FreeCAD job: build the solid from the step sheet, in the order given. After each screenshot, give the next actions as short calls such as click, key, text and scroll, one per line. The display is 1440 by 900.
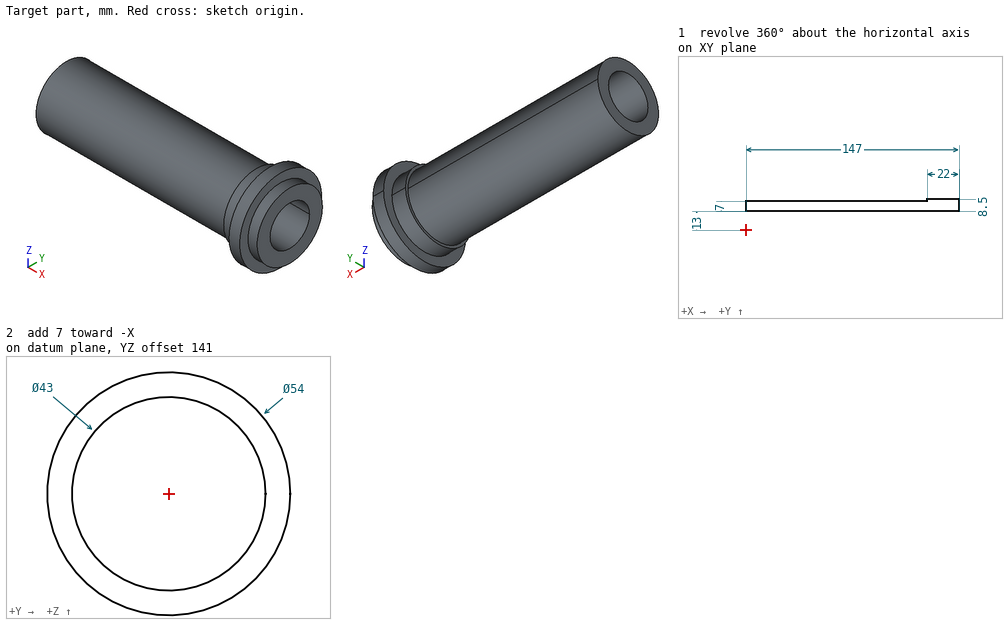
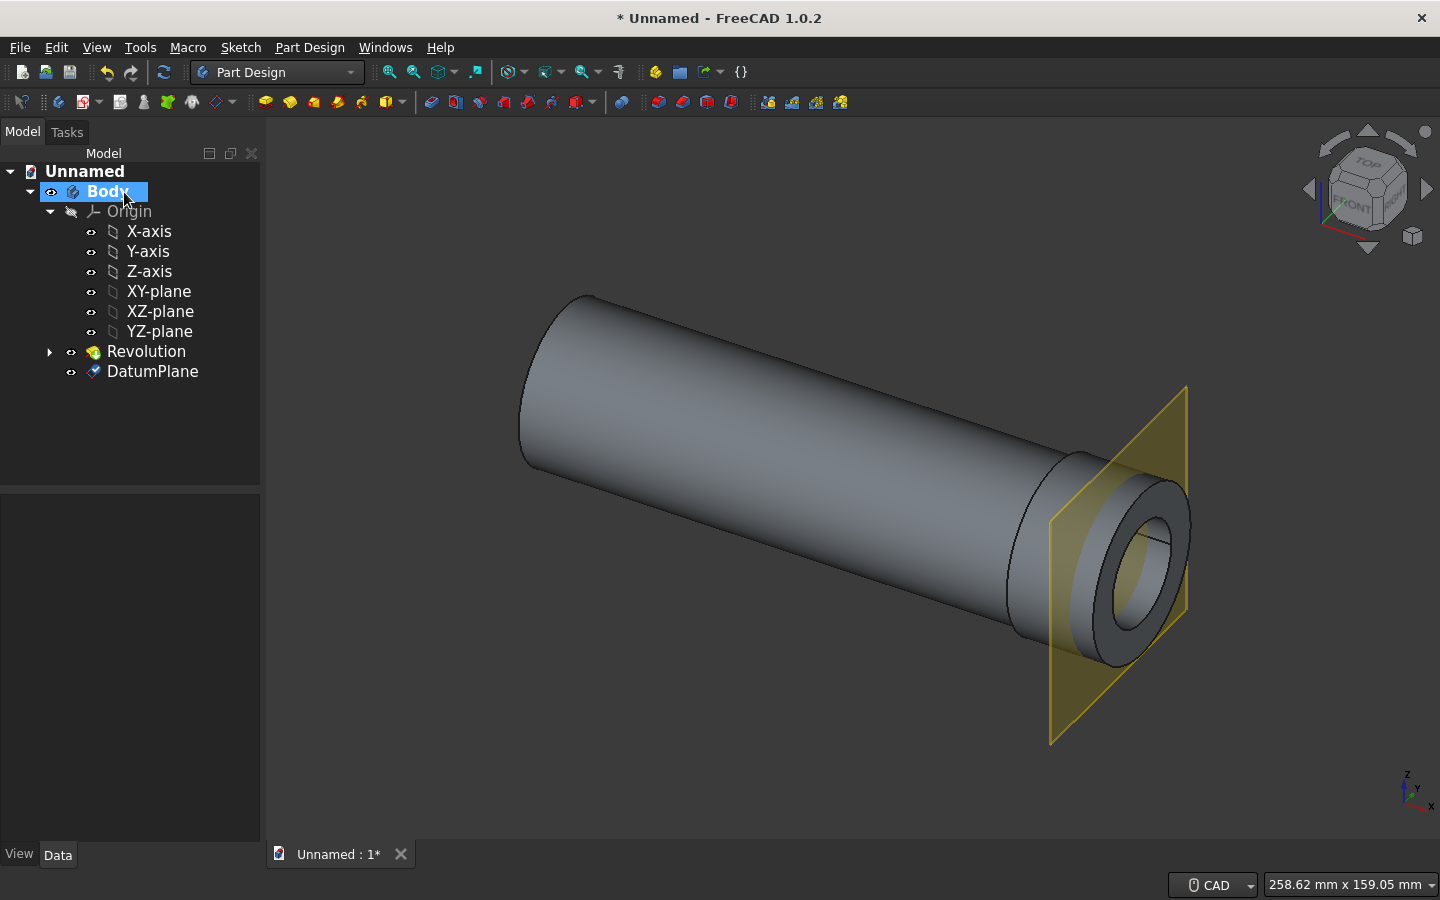
click(116, 372)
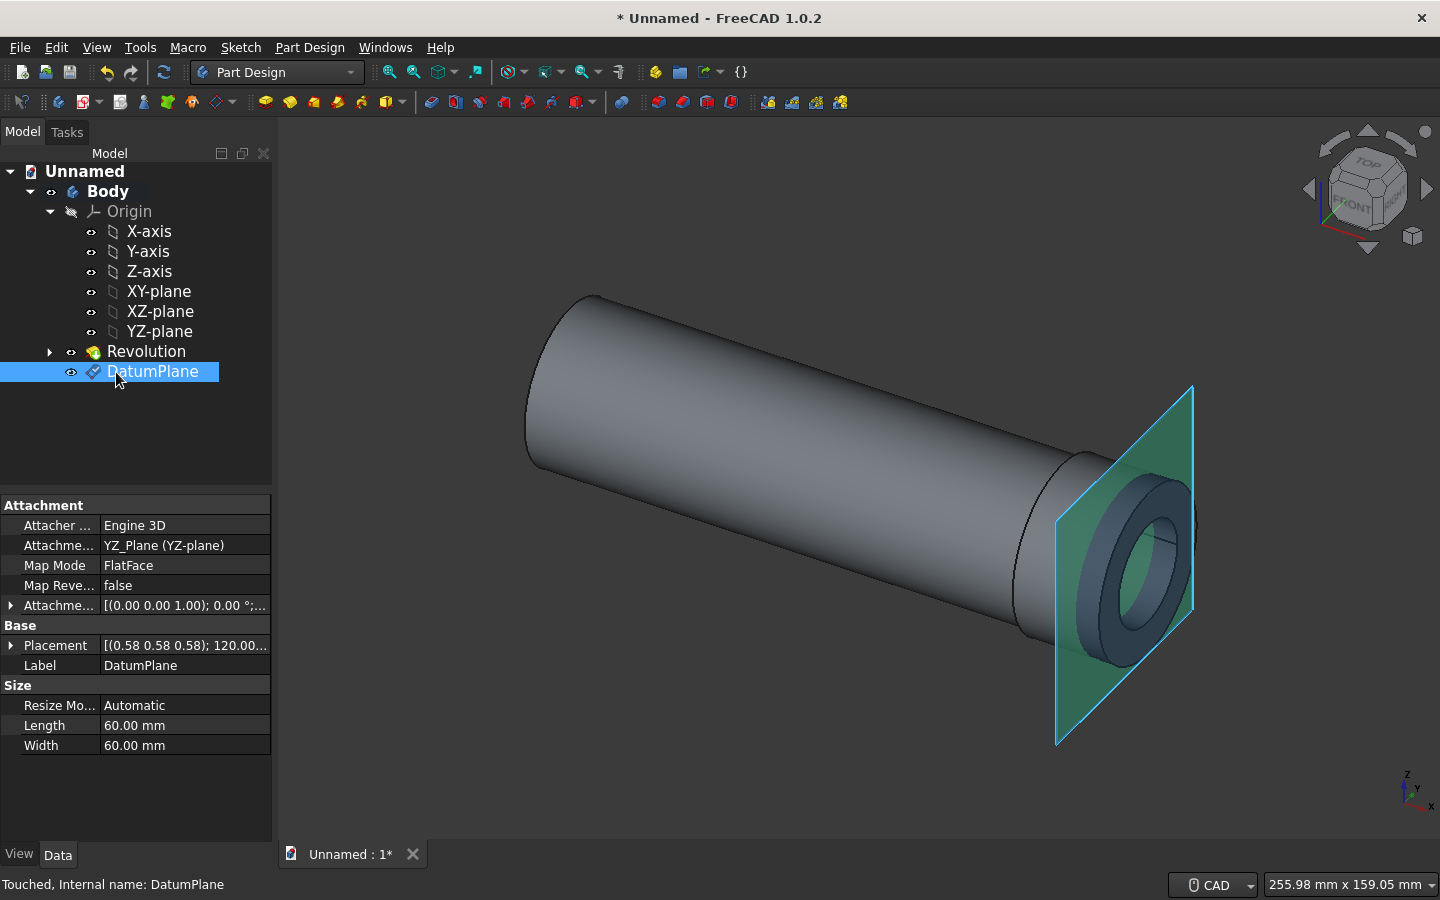
click(84, 102)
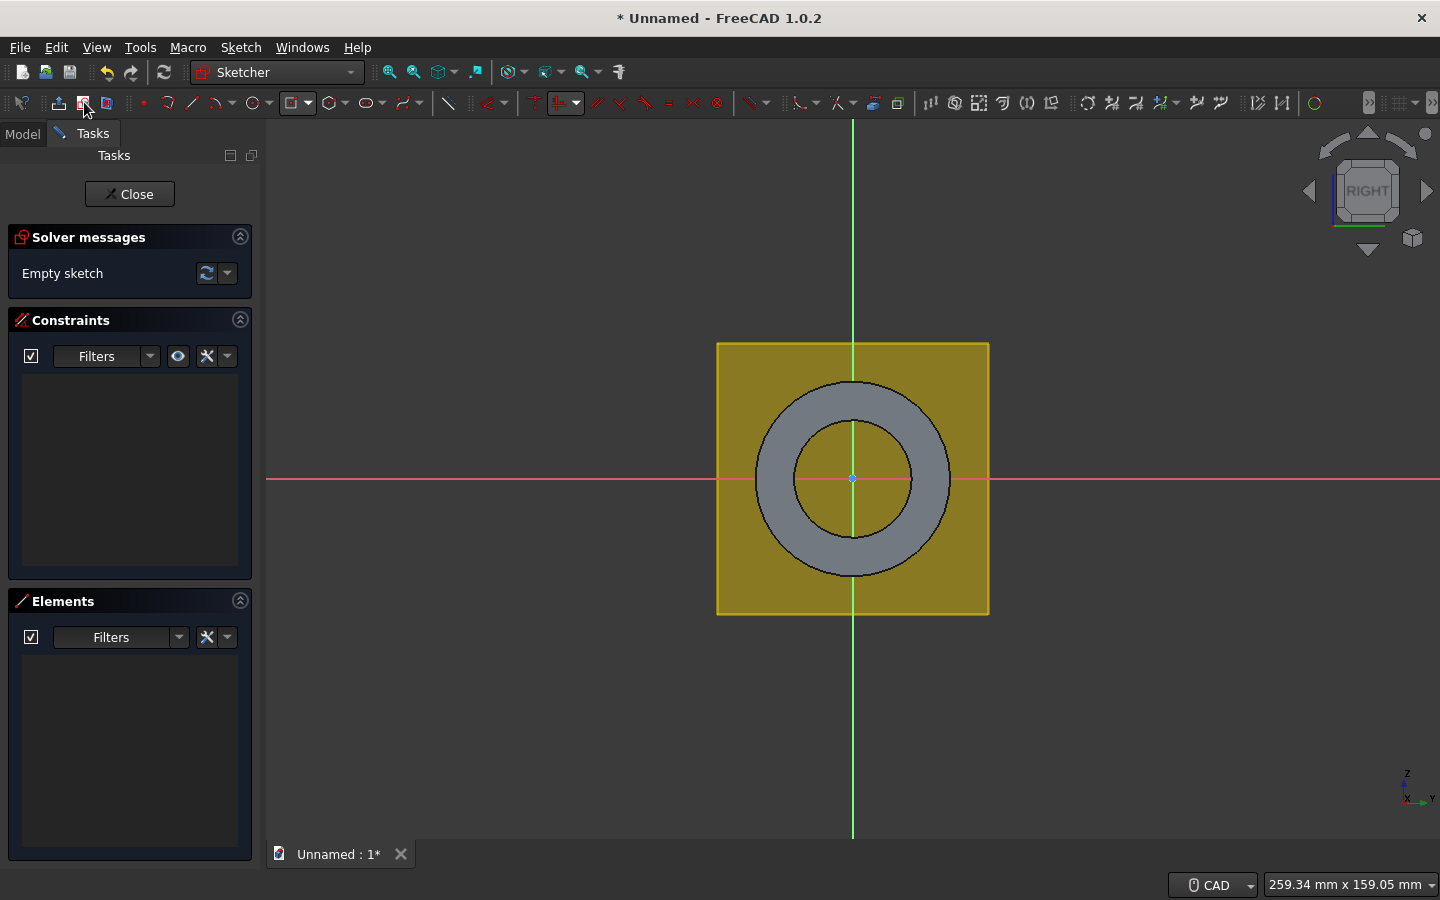
click(108, 104)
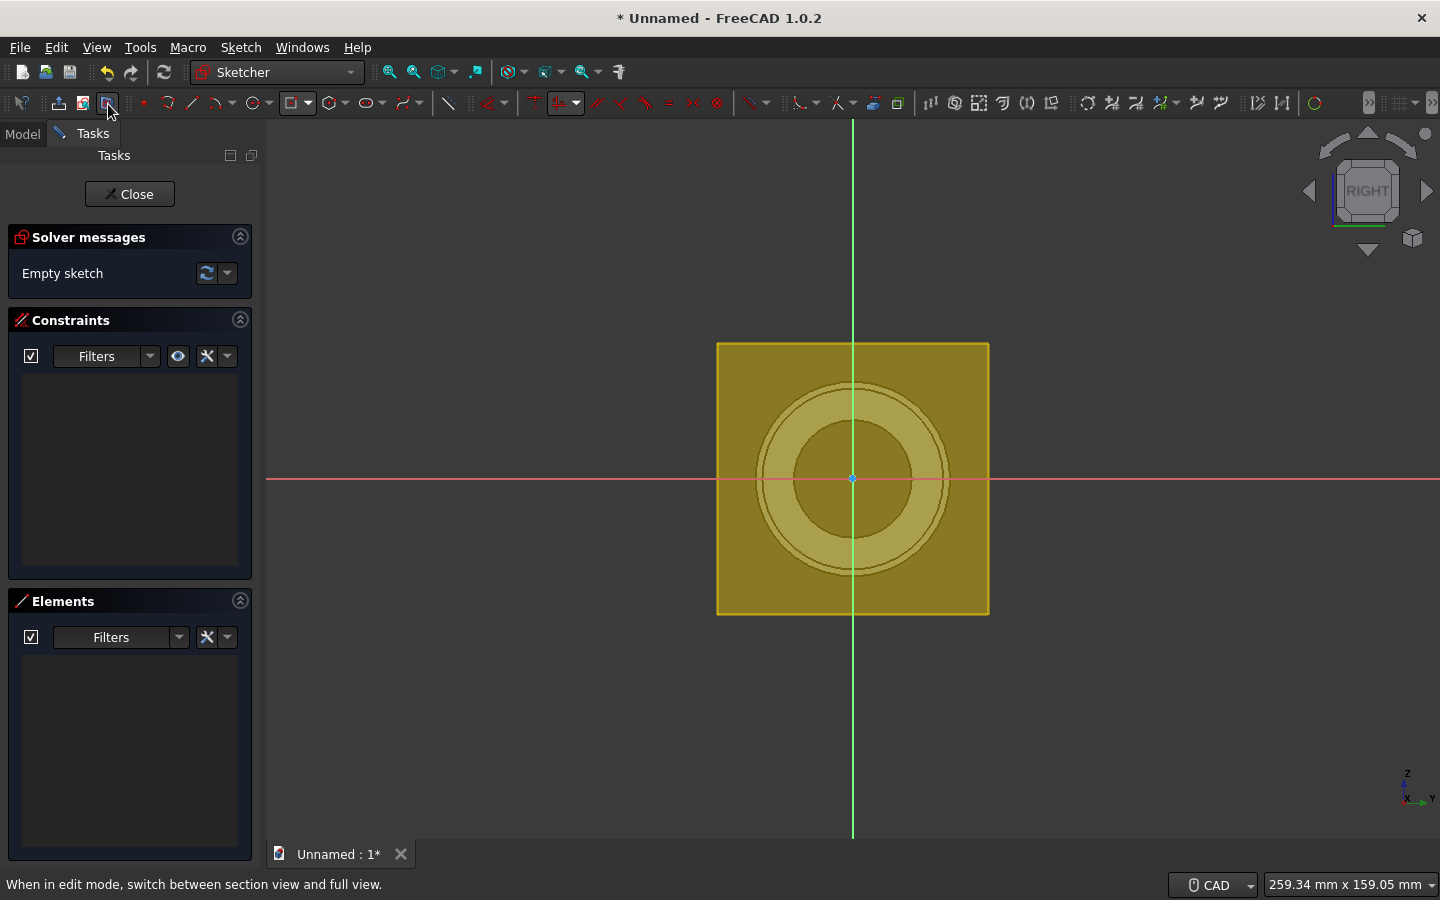
scroll(936, 479, up, 3)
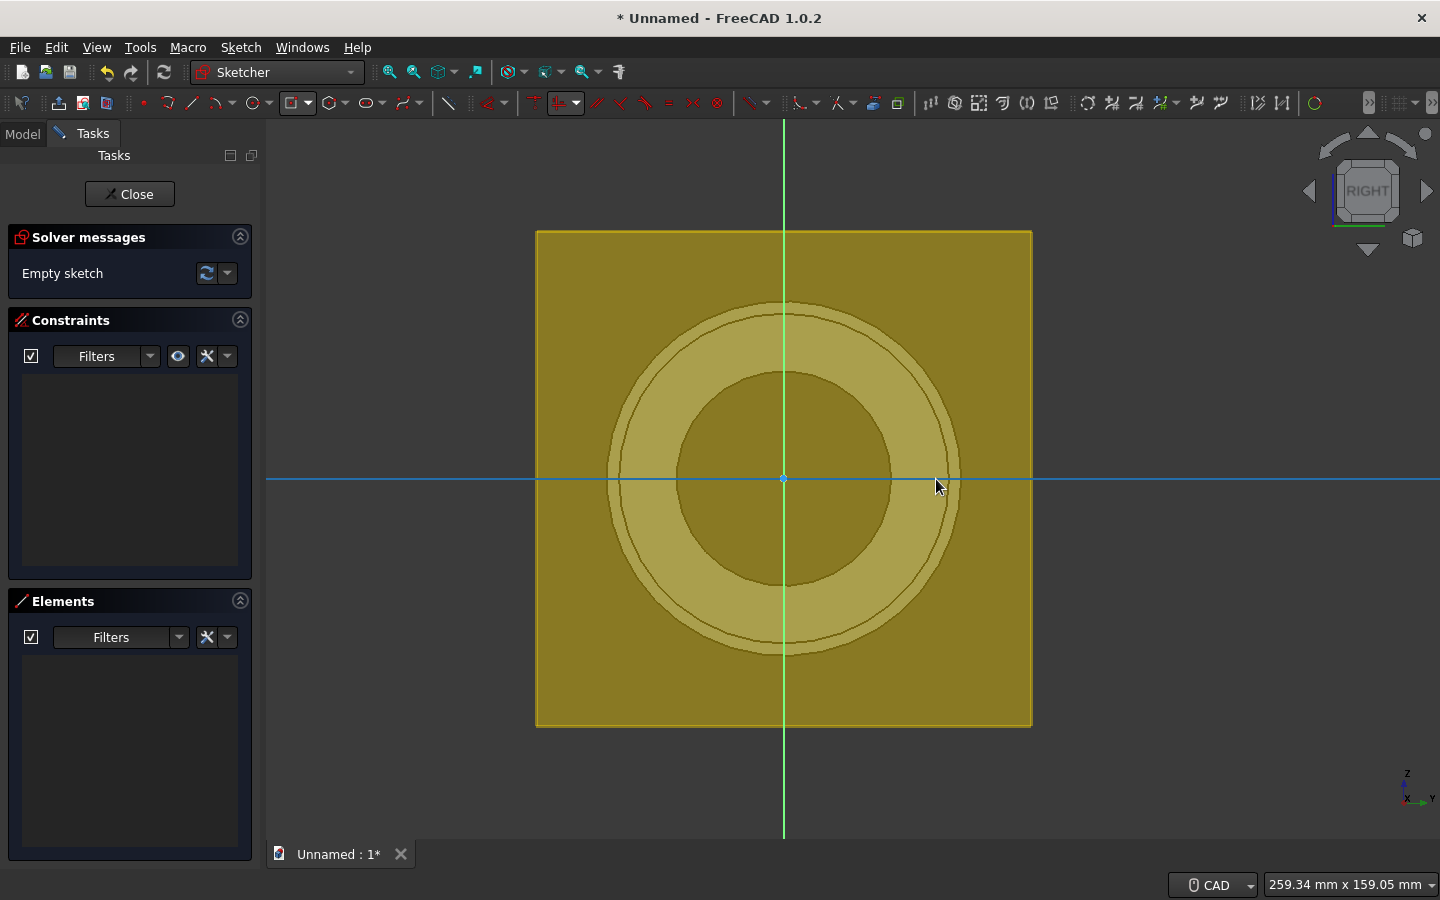
click(254, 104)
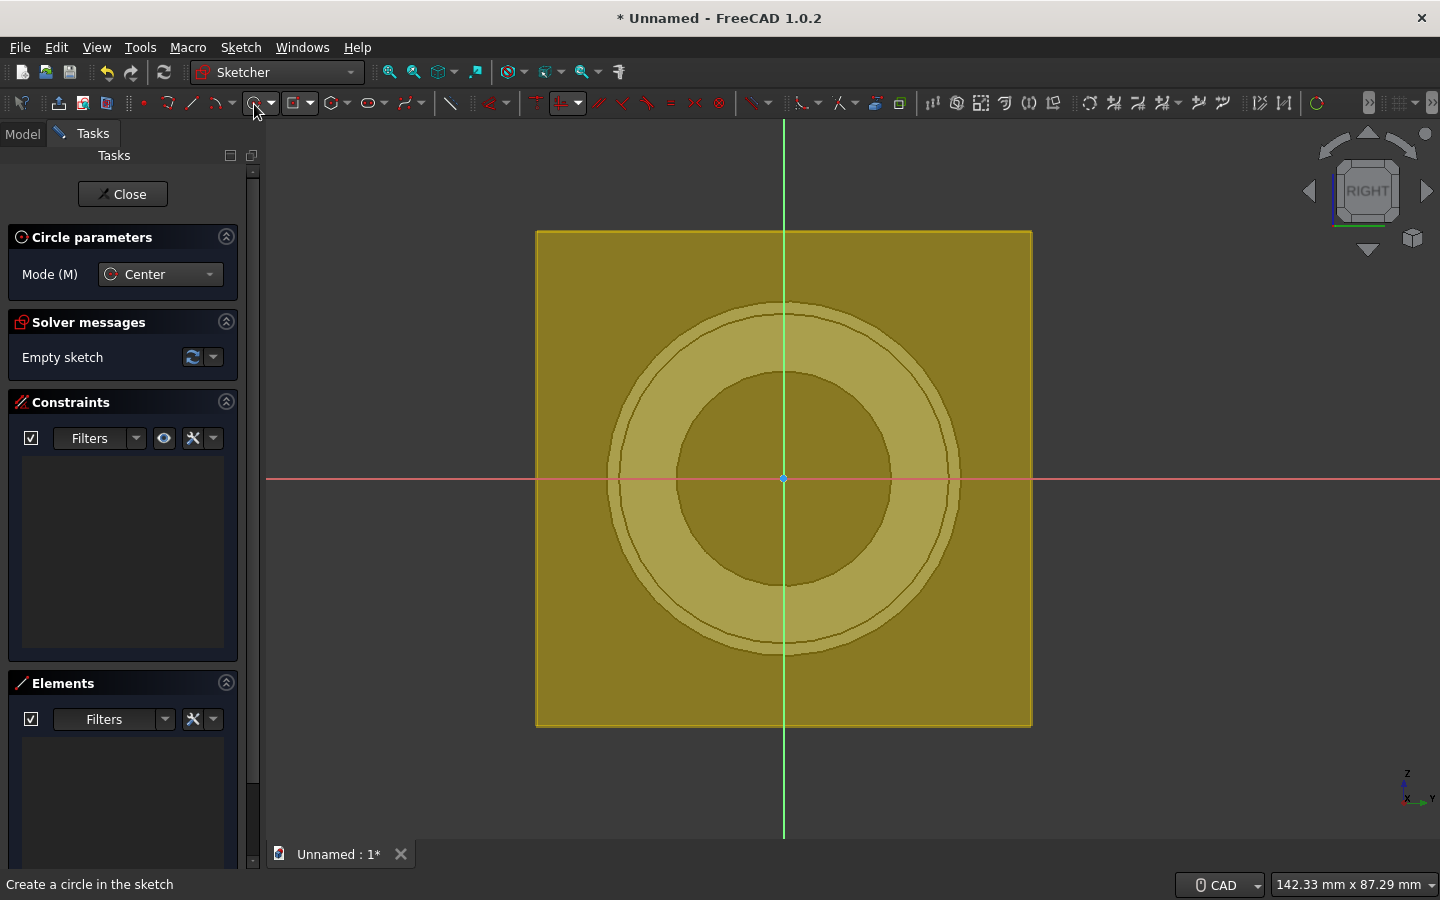
click(784, 479)
click(941, 321)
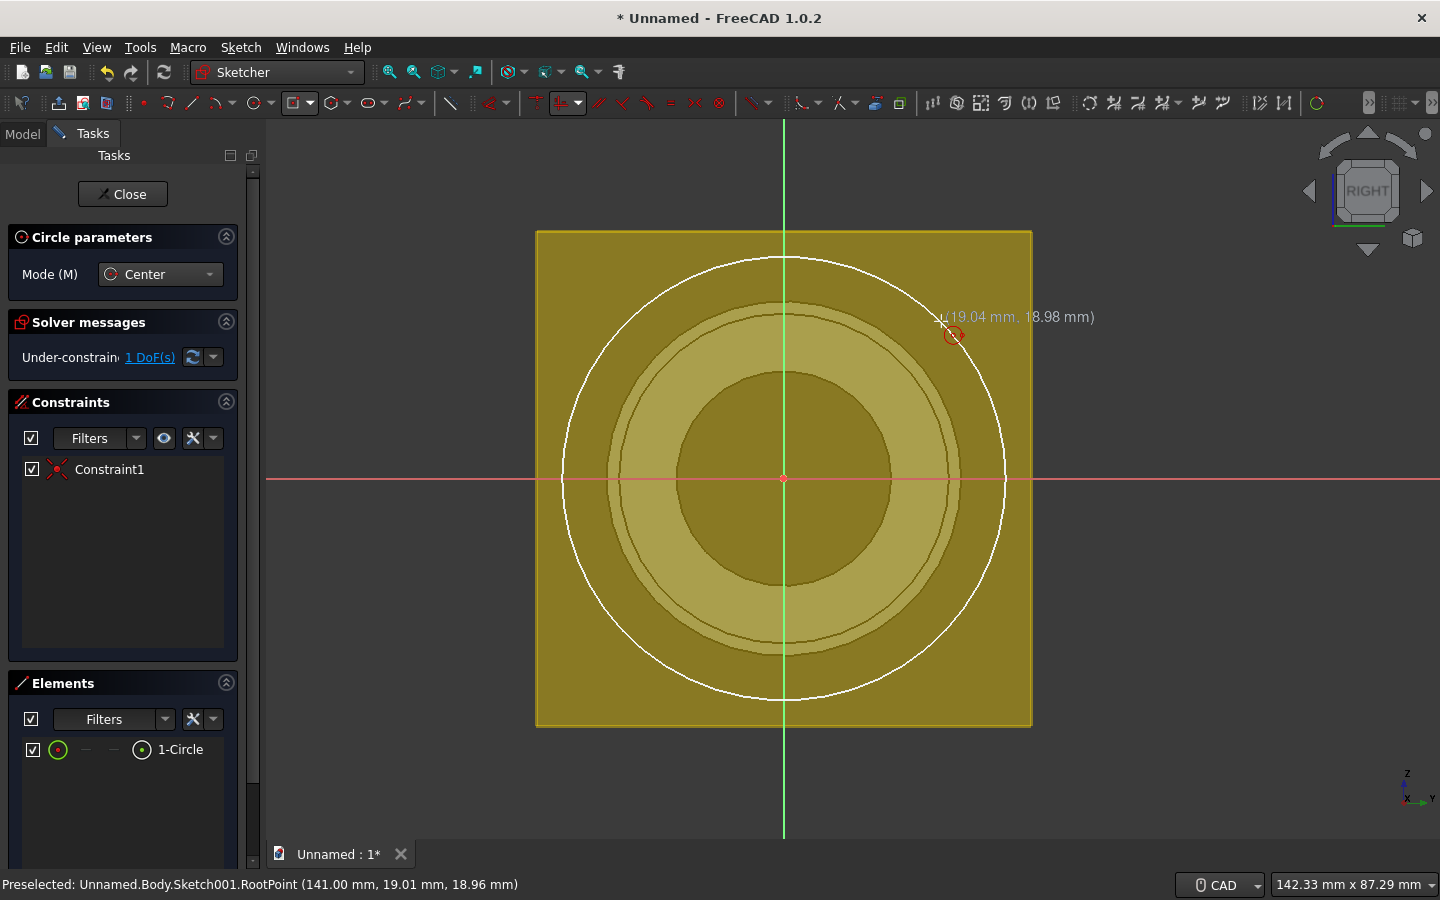
click(784, 479)
click(909, 353)
key(Escape)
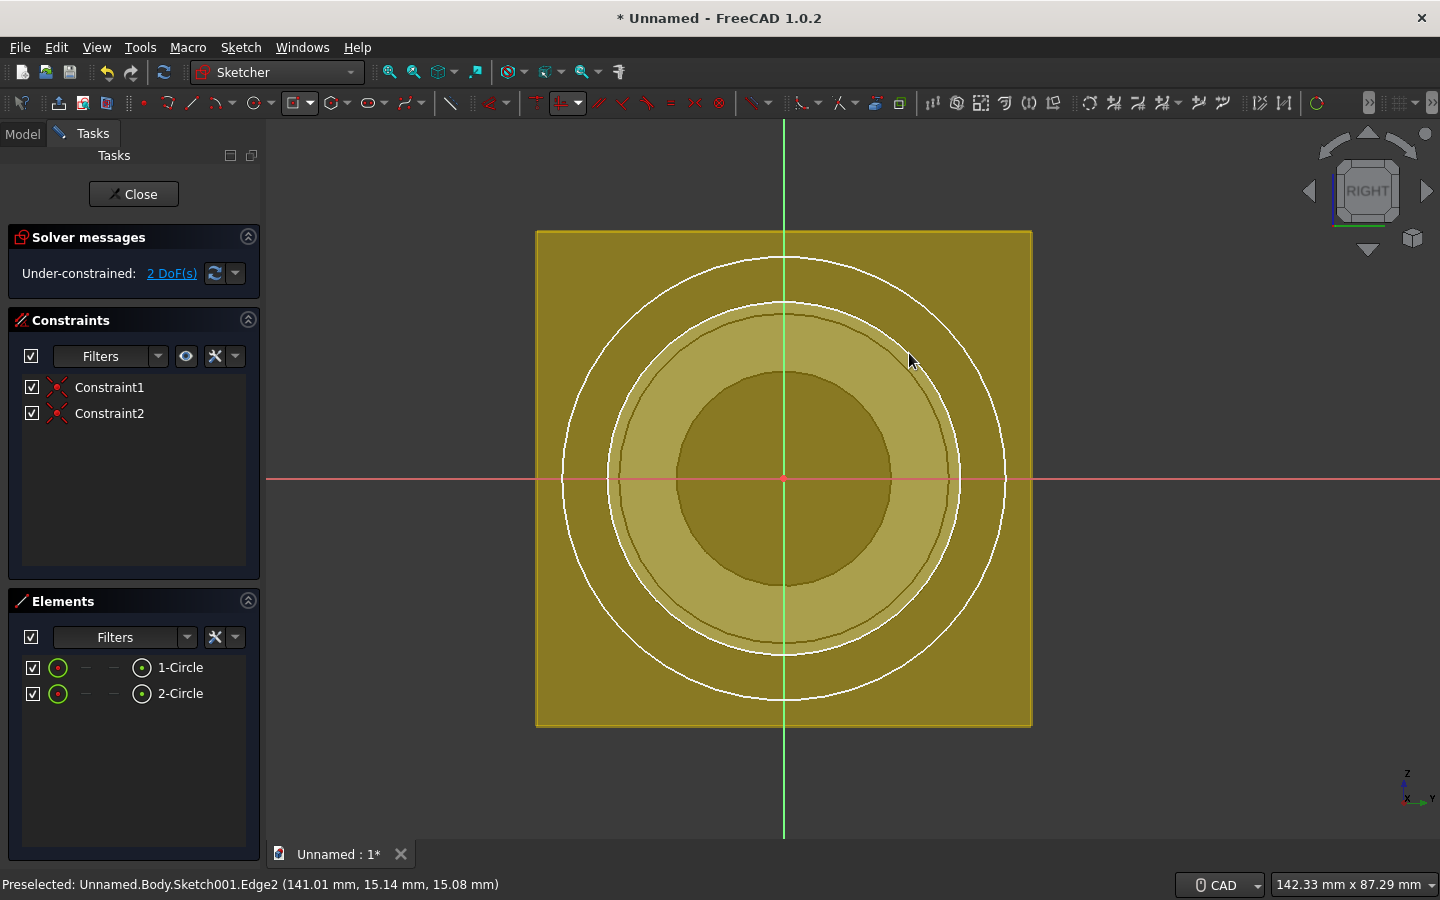
click(490, 104)